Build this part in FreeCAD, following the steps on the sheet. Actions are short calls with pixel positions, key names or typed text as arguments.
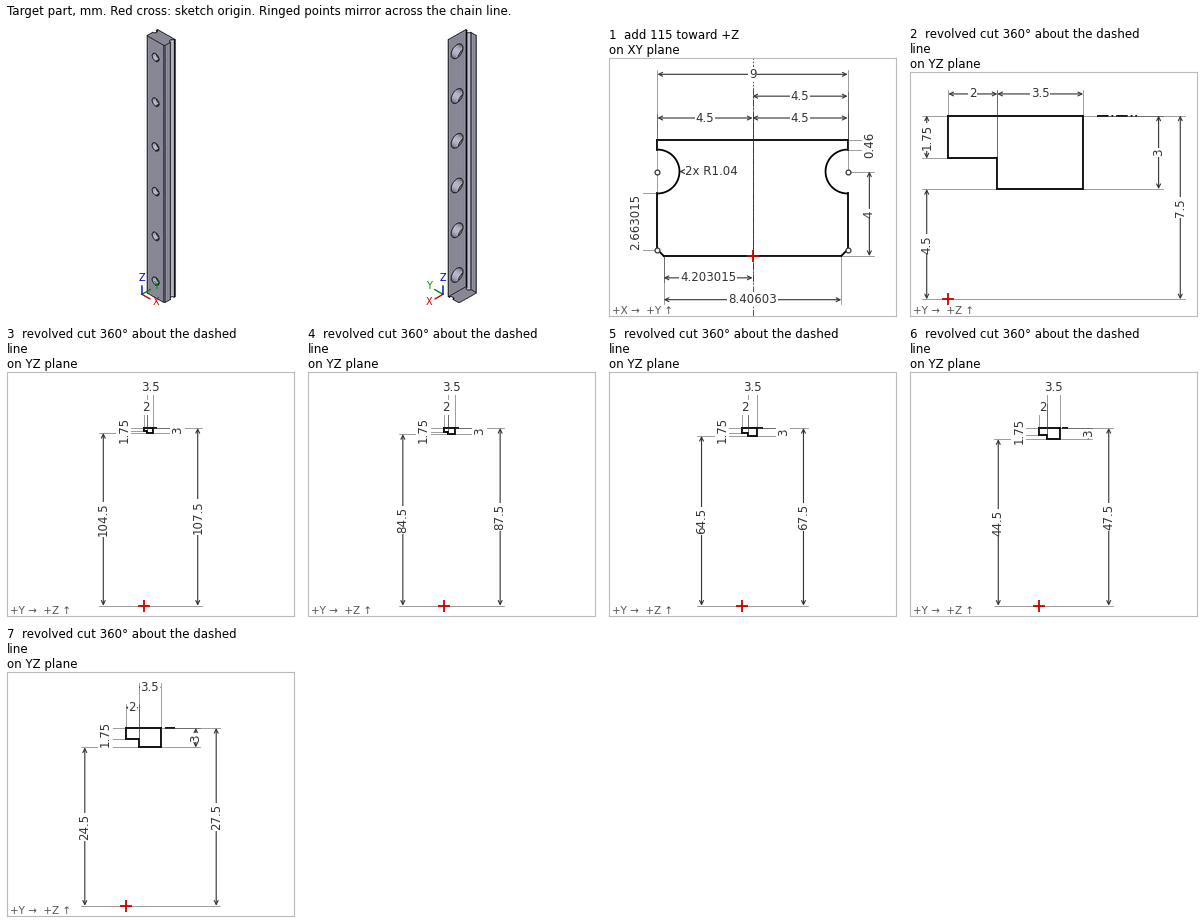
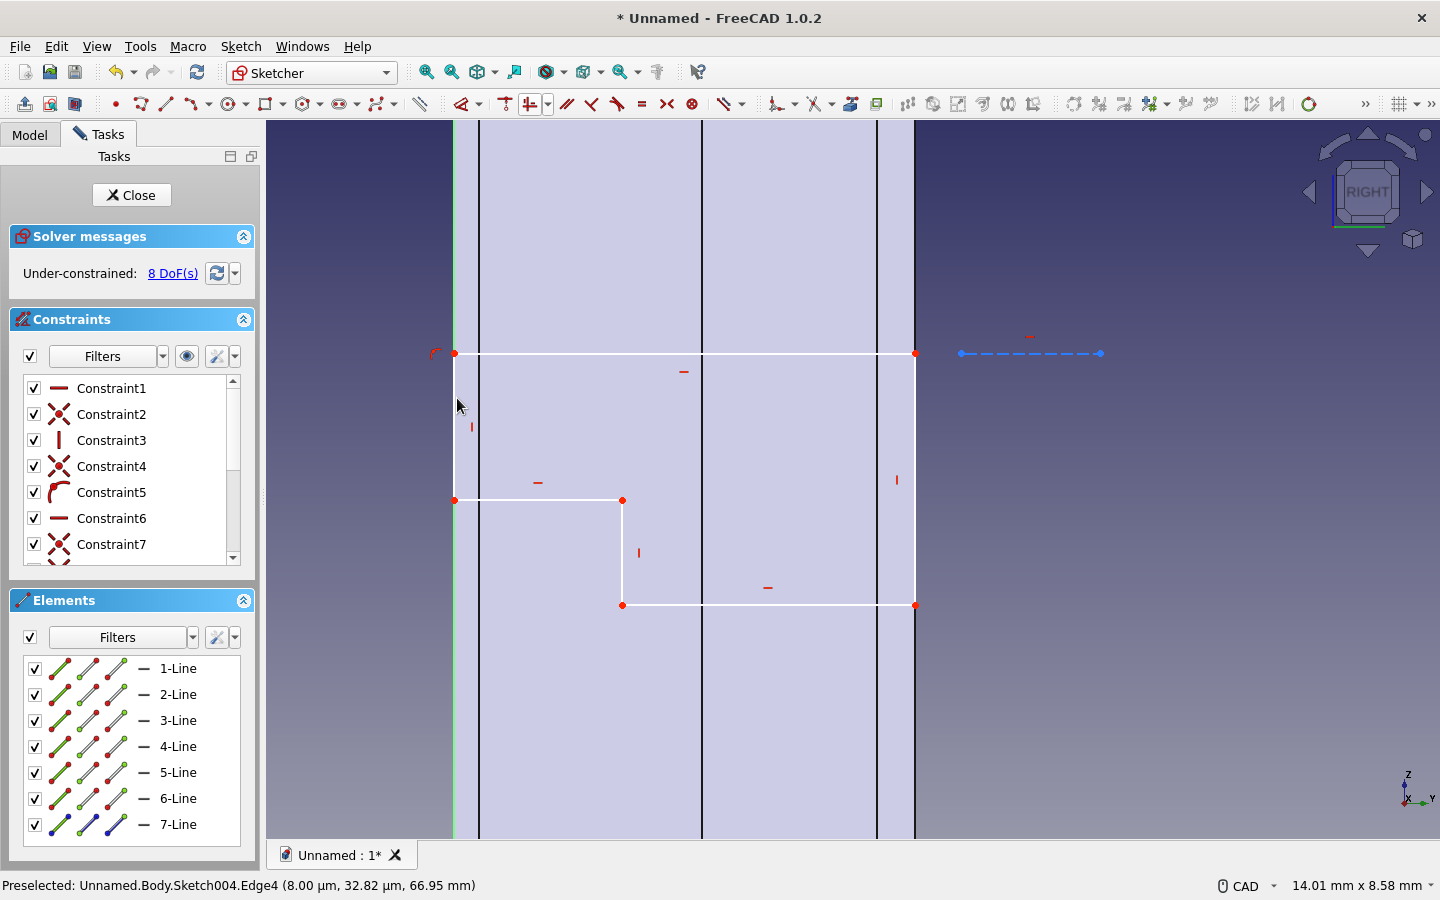
key(d)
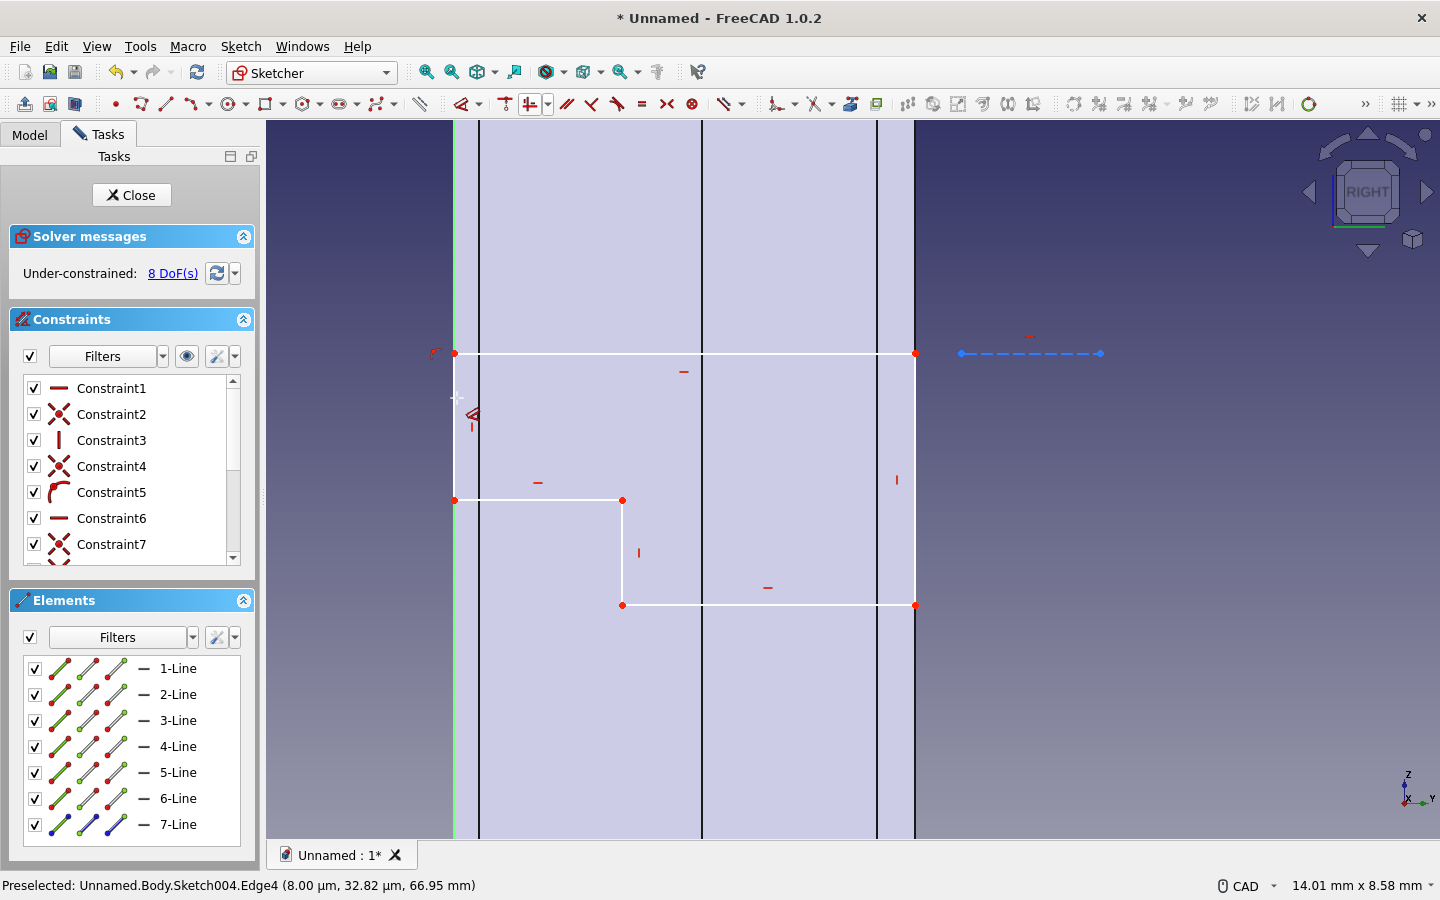
click(915, 530)
click(949, 480)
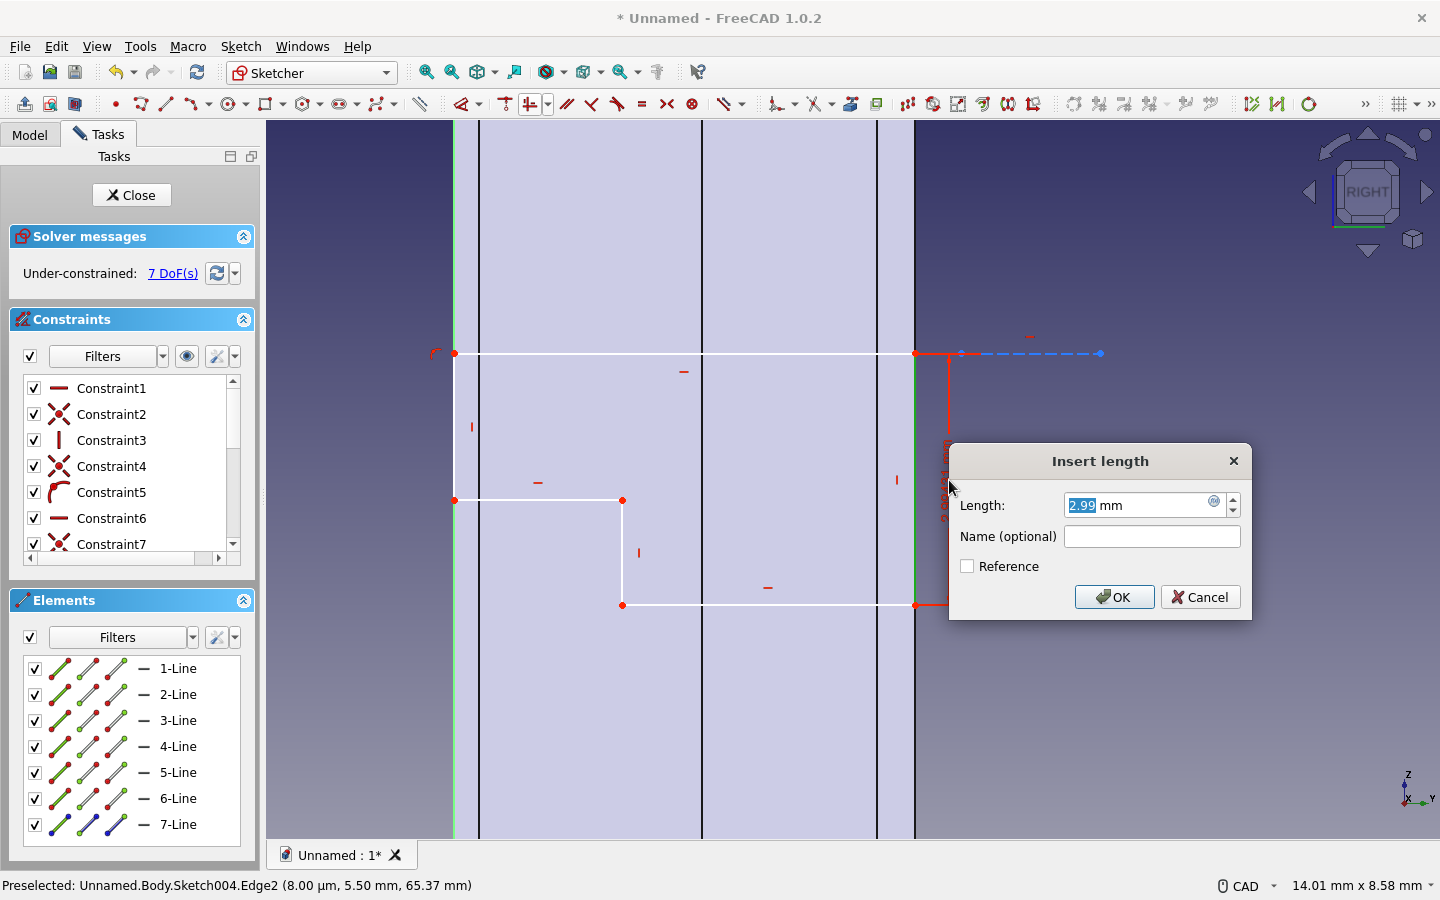
text(3)
key(Return)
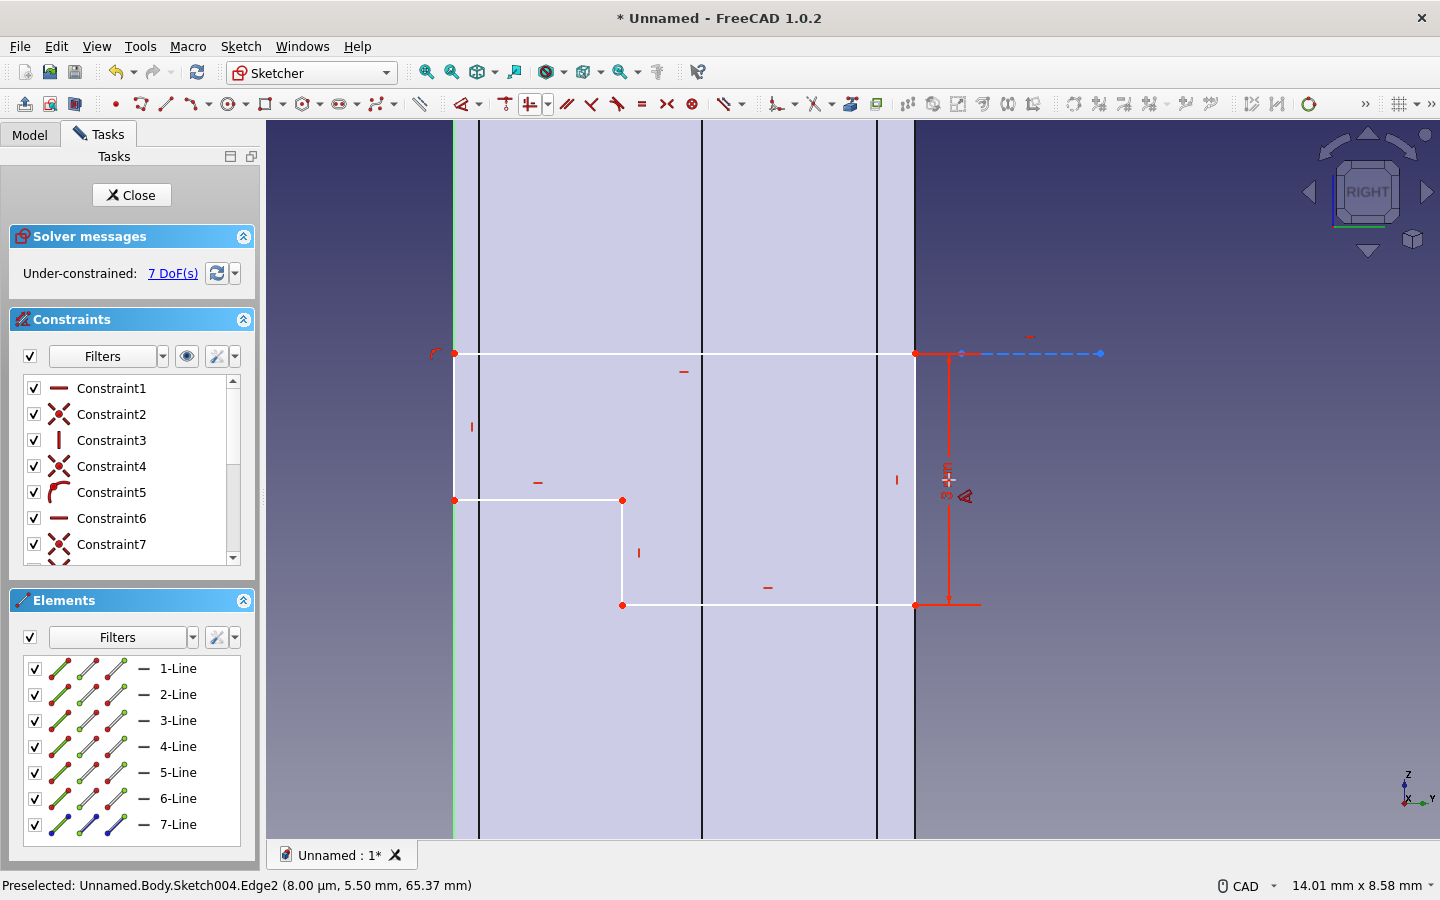
click(504, 500)
click(538, 534)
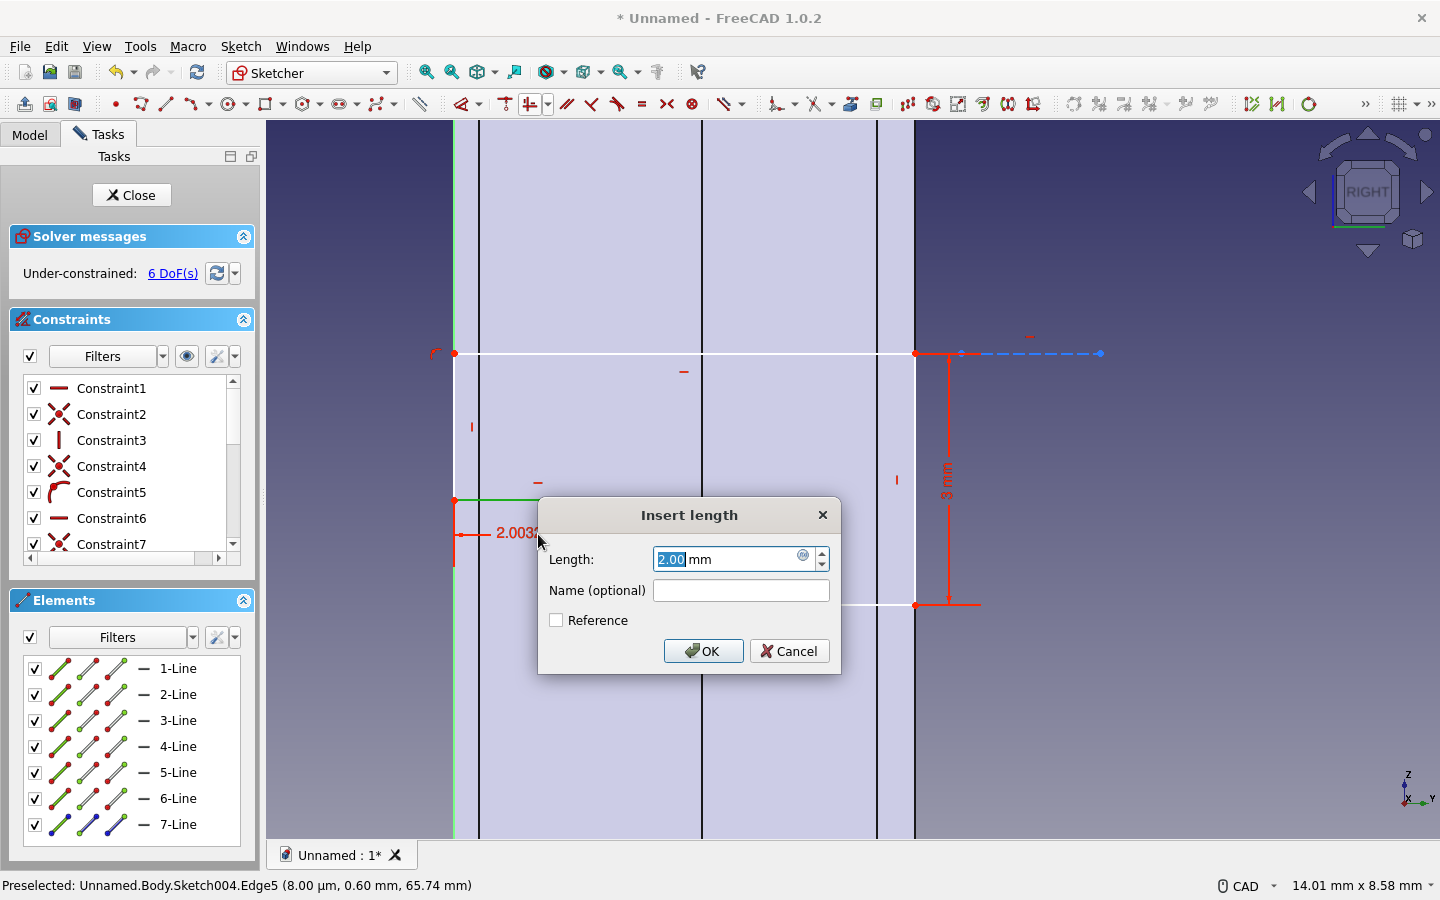
text(2)
key(Return)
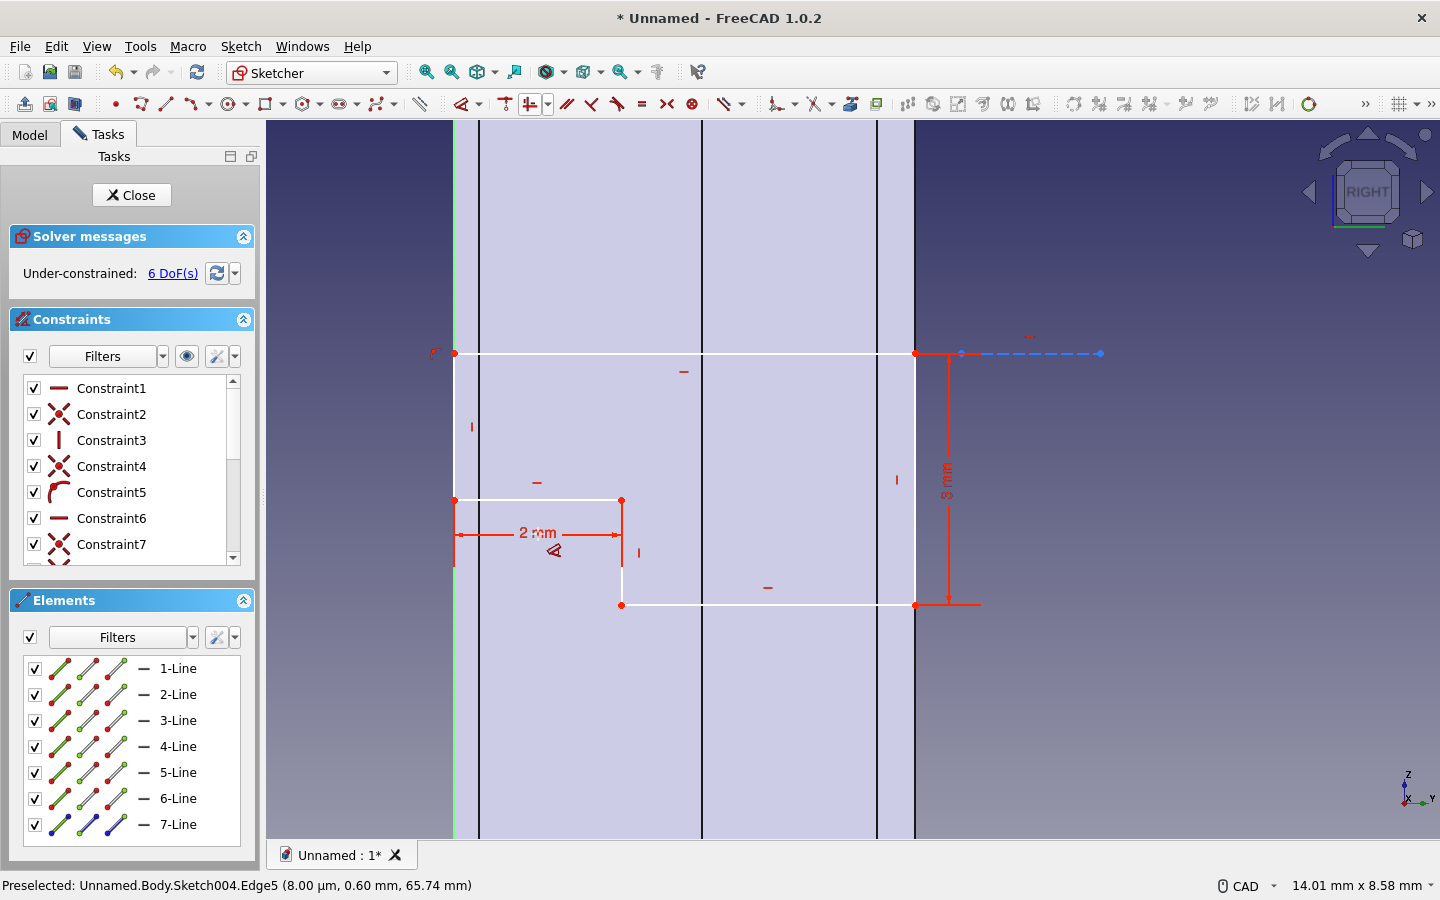
click(710, 605)
click(768, 639)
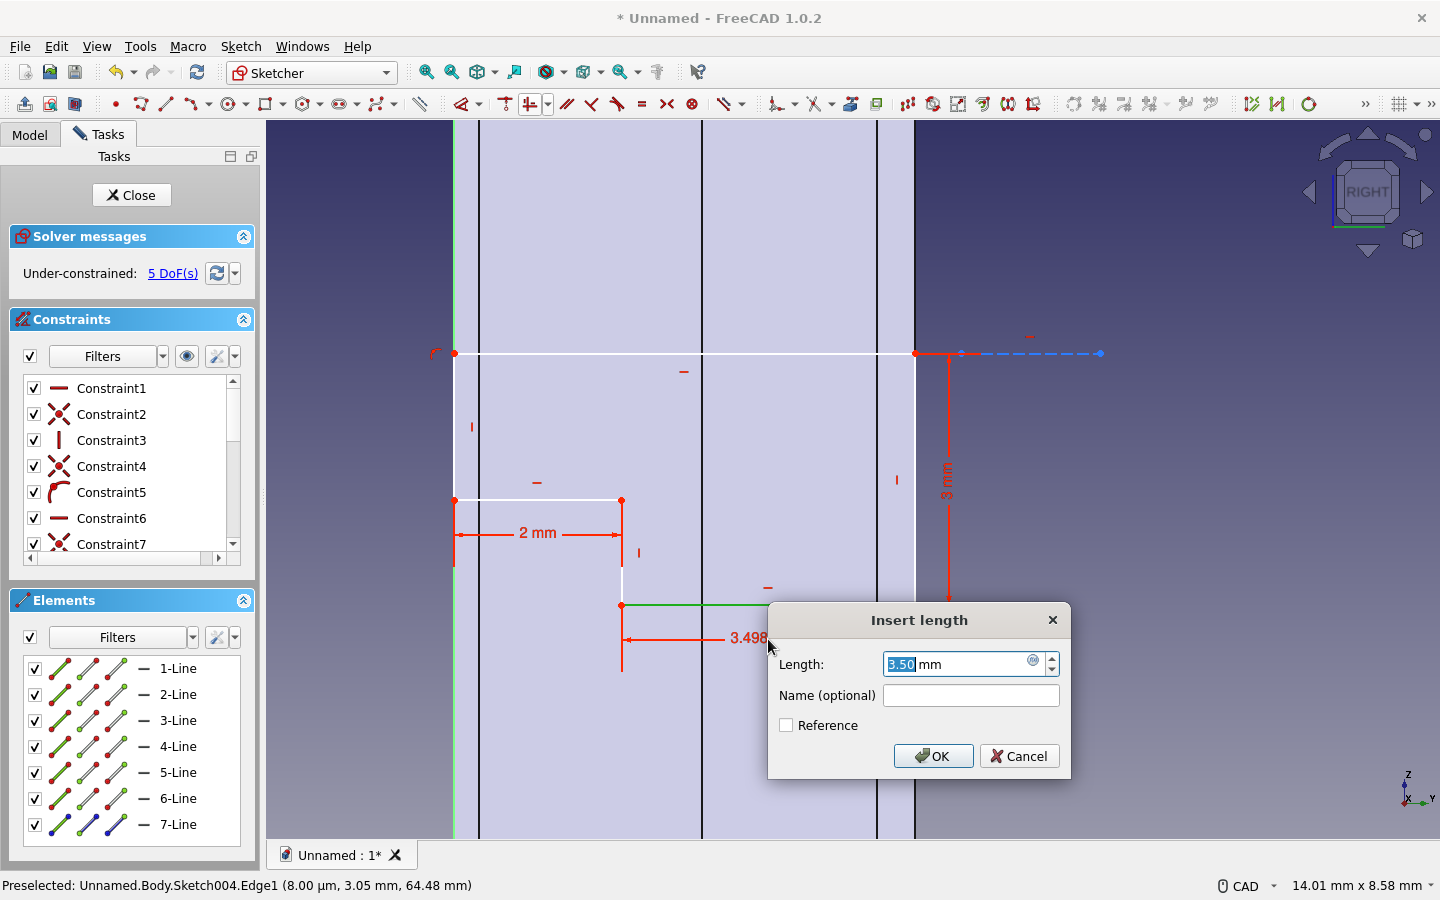
text(3.5)
key(Return)